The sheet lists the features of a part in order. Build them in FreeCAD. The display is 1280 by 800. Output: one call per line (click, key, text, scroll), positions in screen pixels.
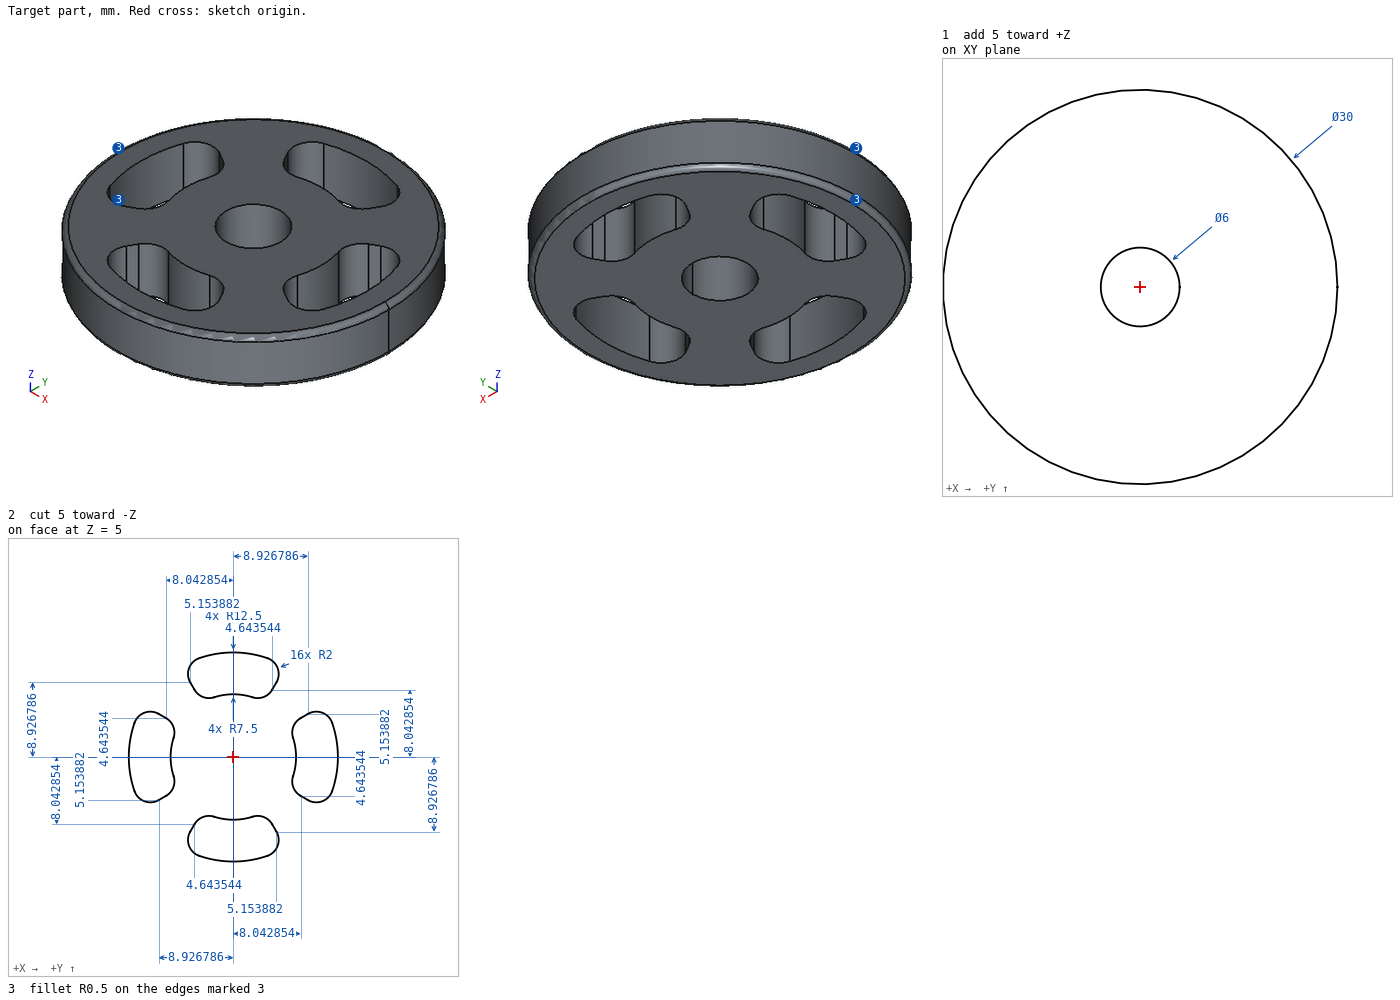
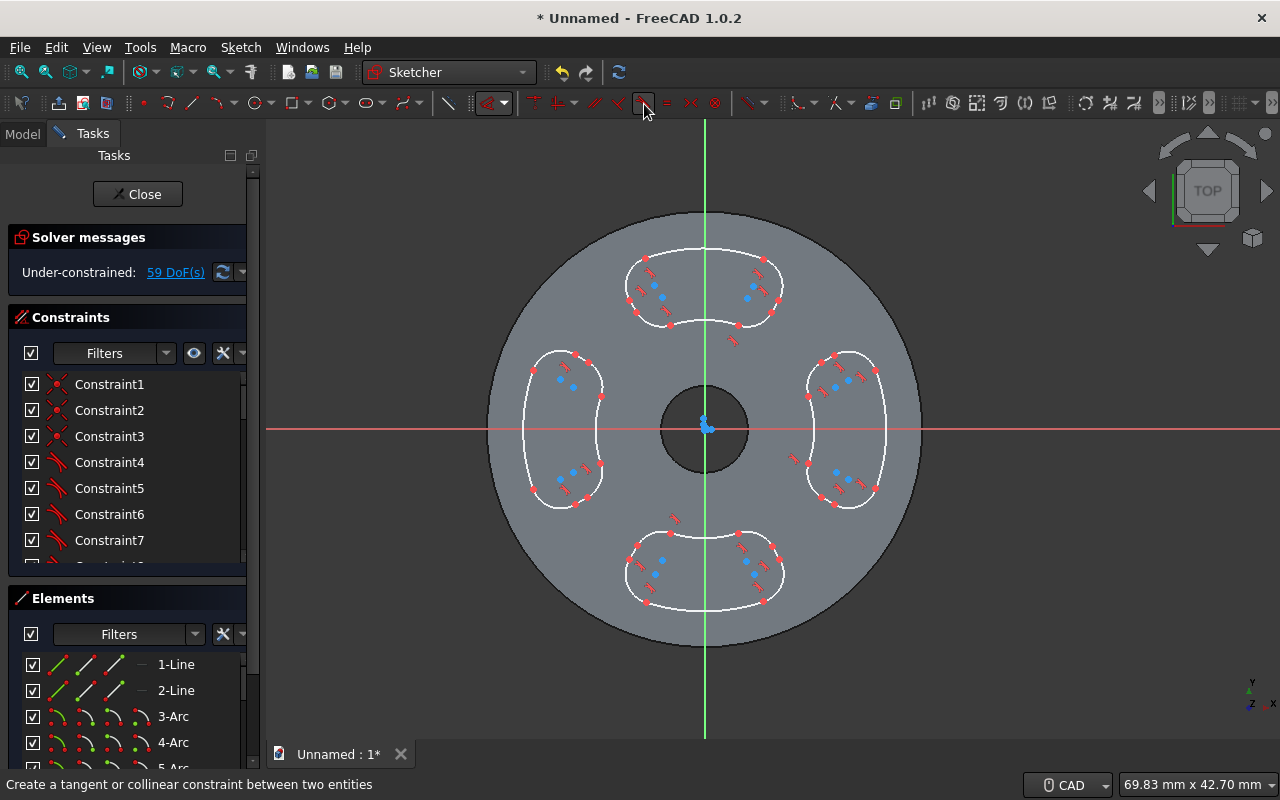
click(597, 416)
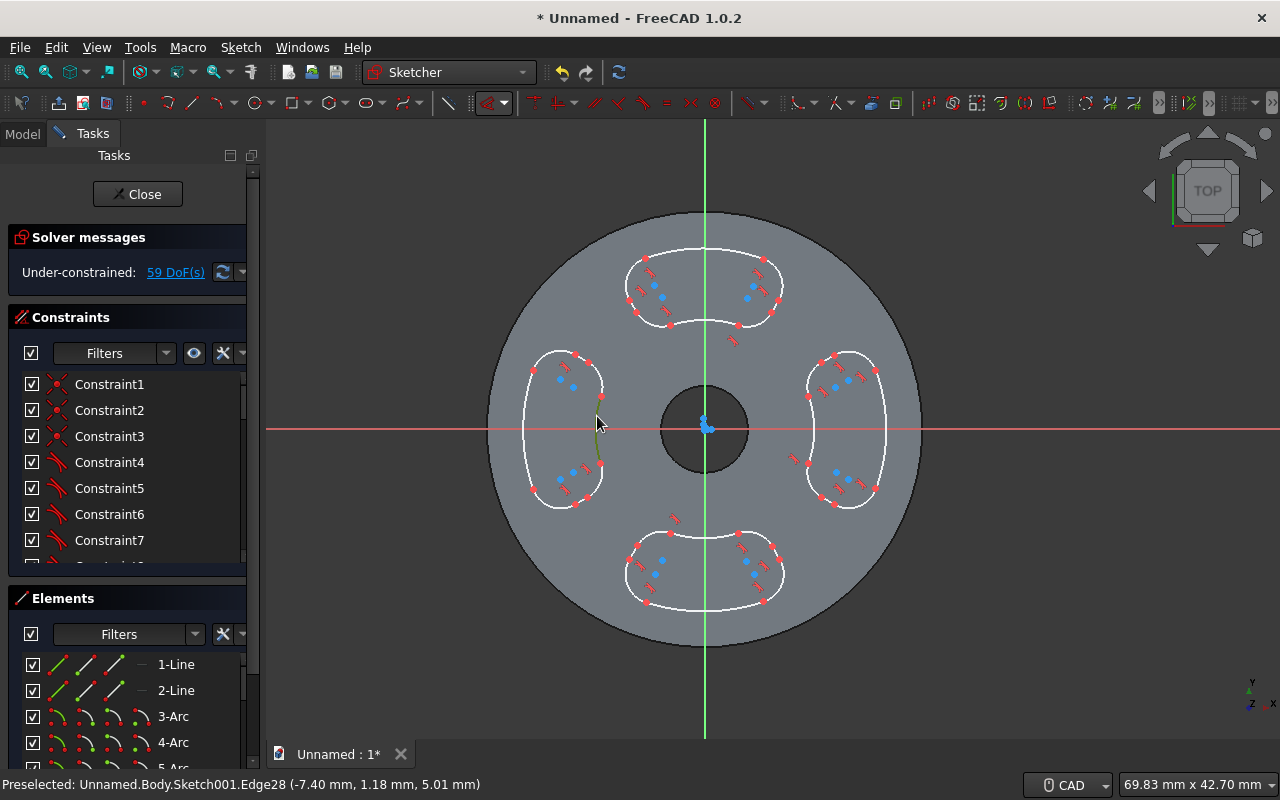
click(602, 385)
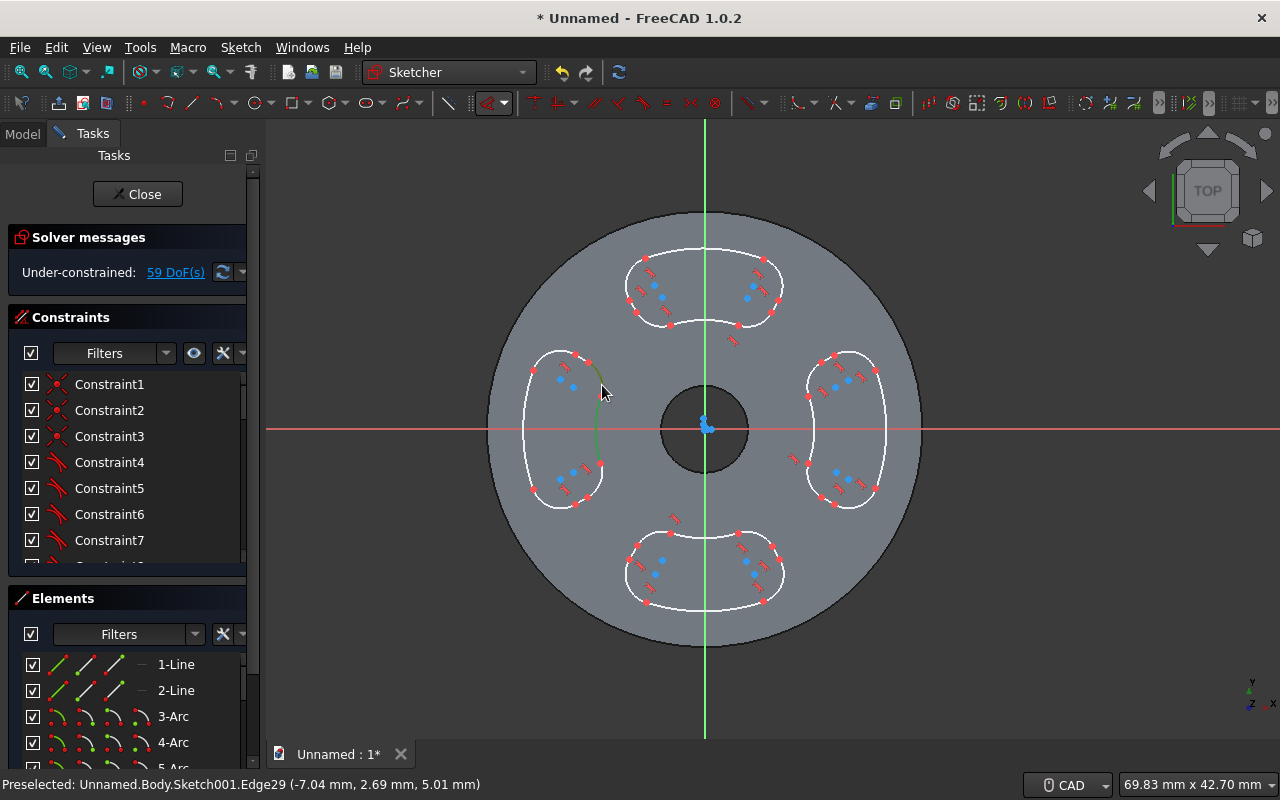
click(644, 104)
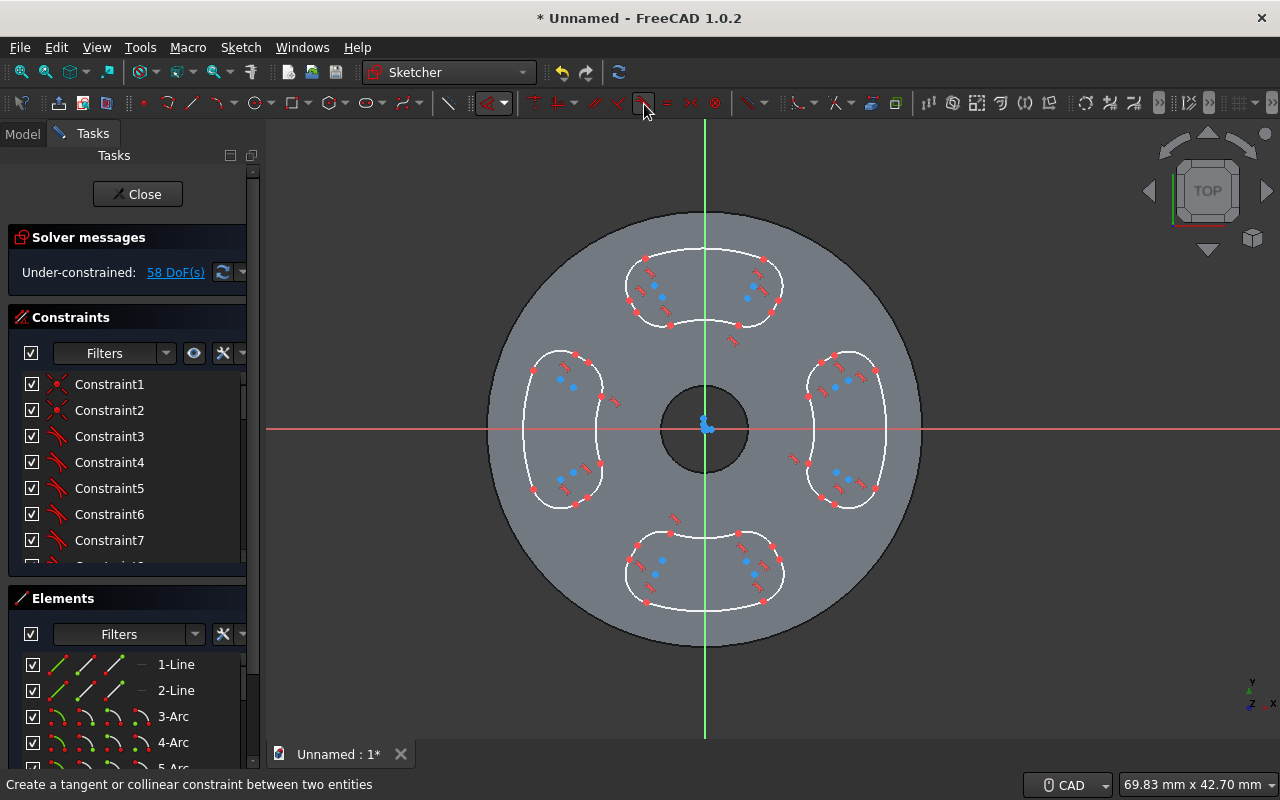
click(560, 351)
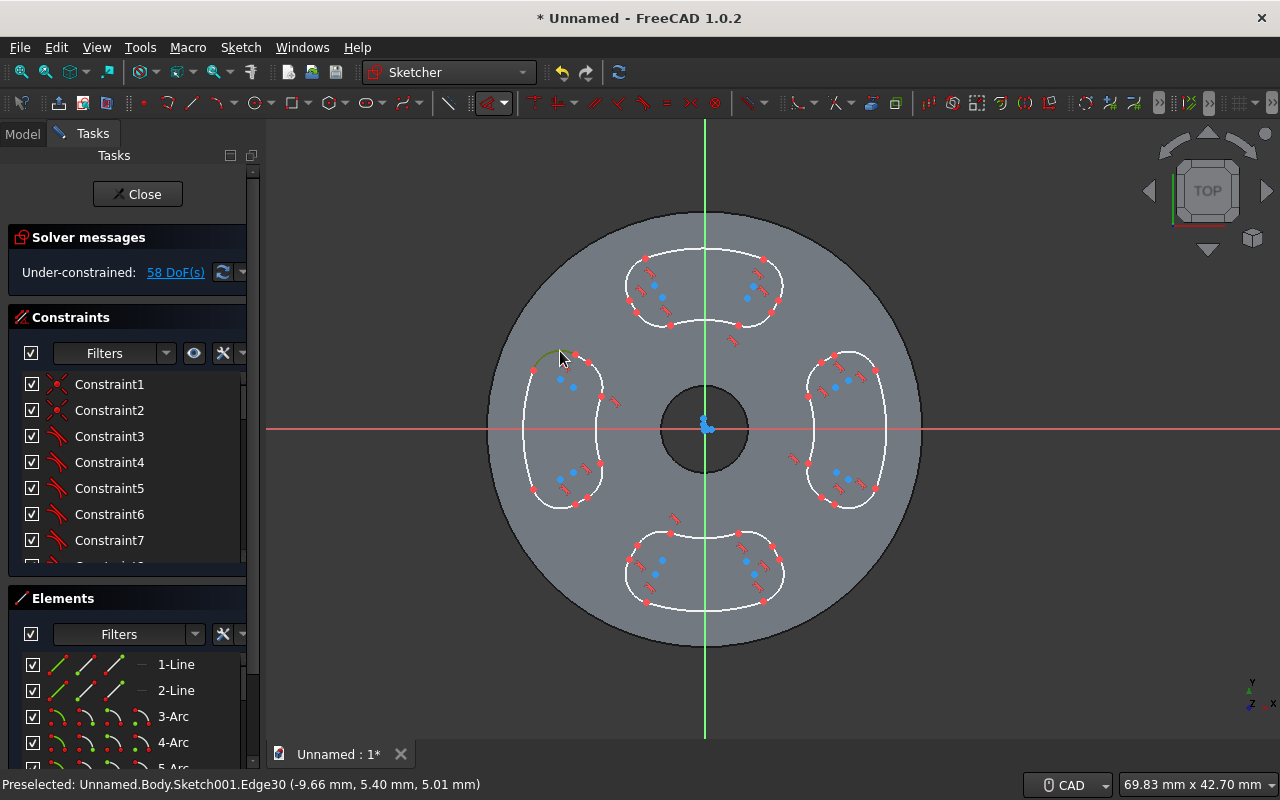
click(525, 406)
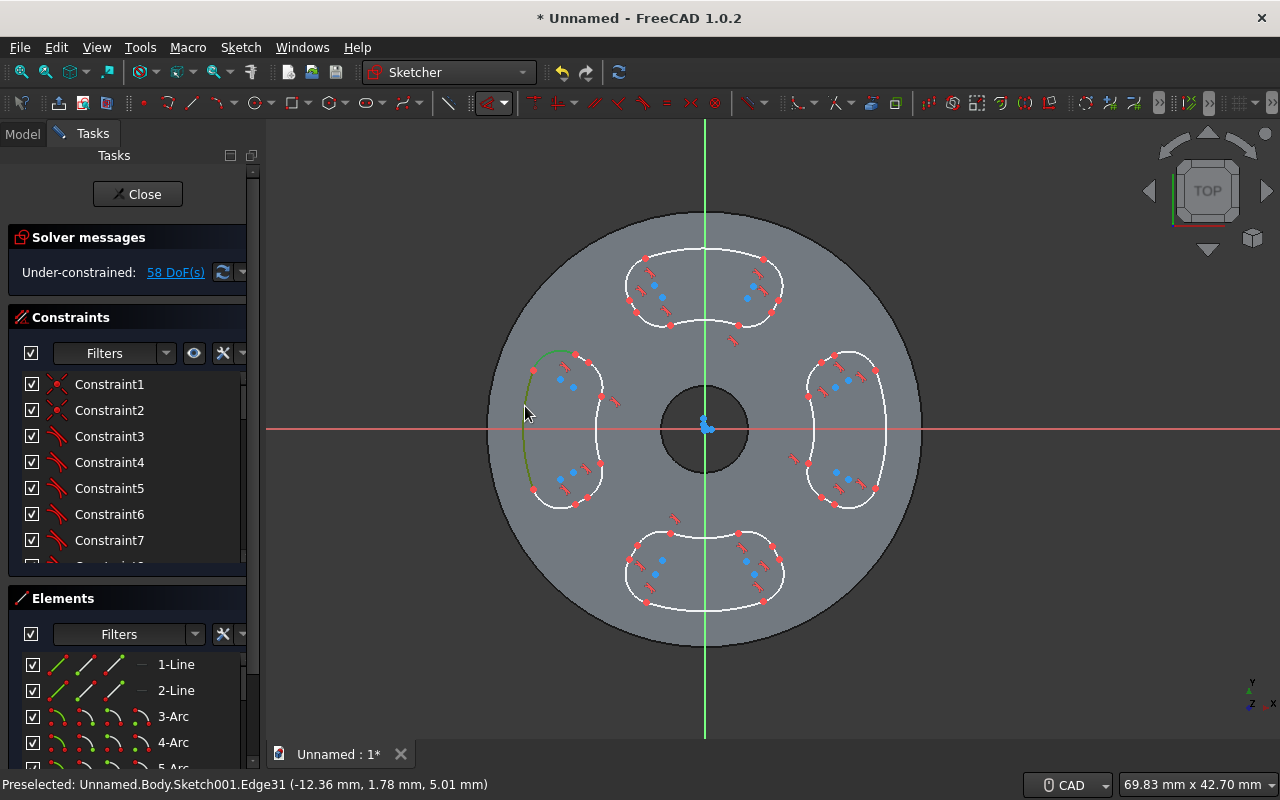
click(644, 104)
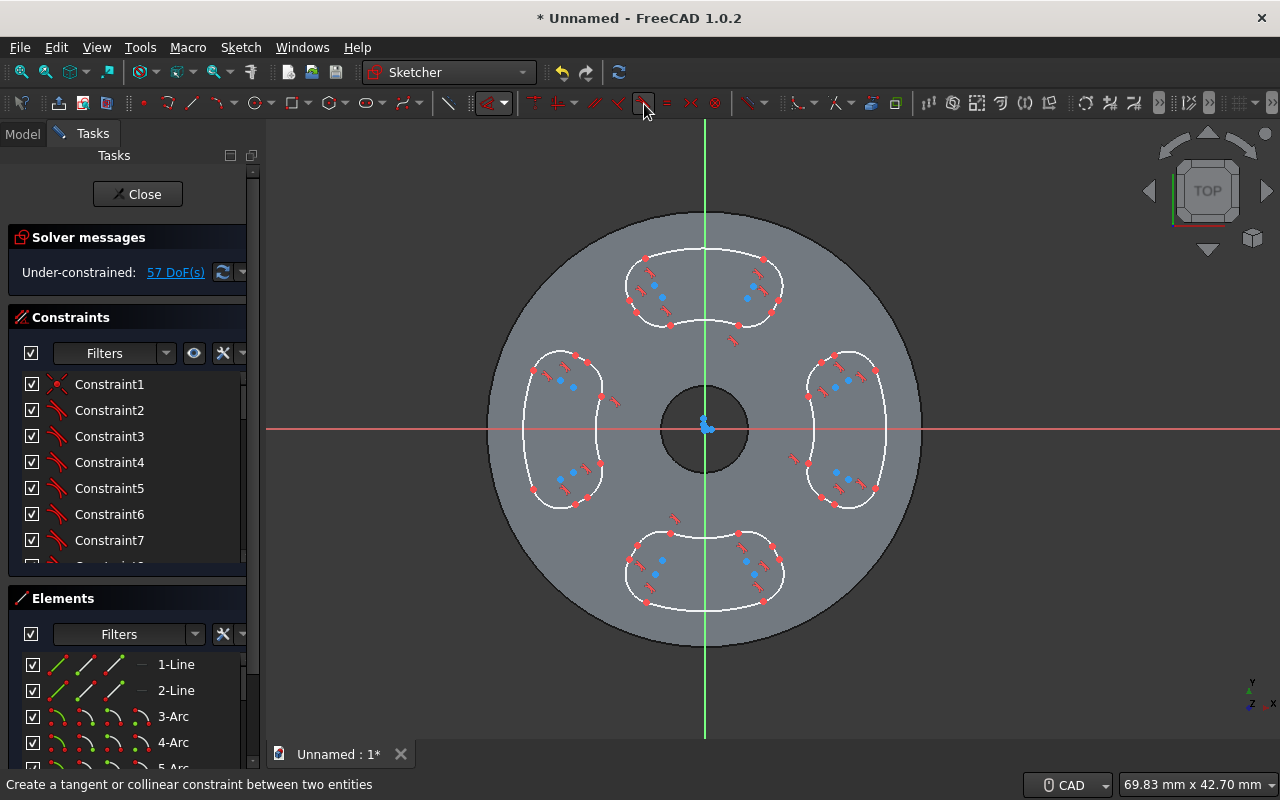
click(525, 406)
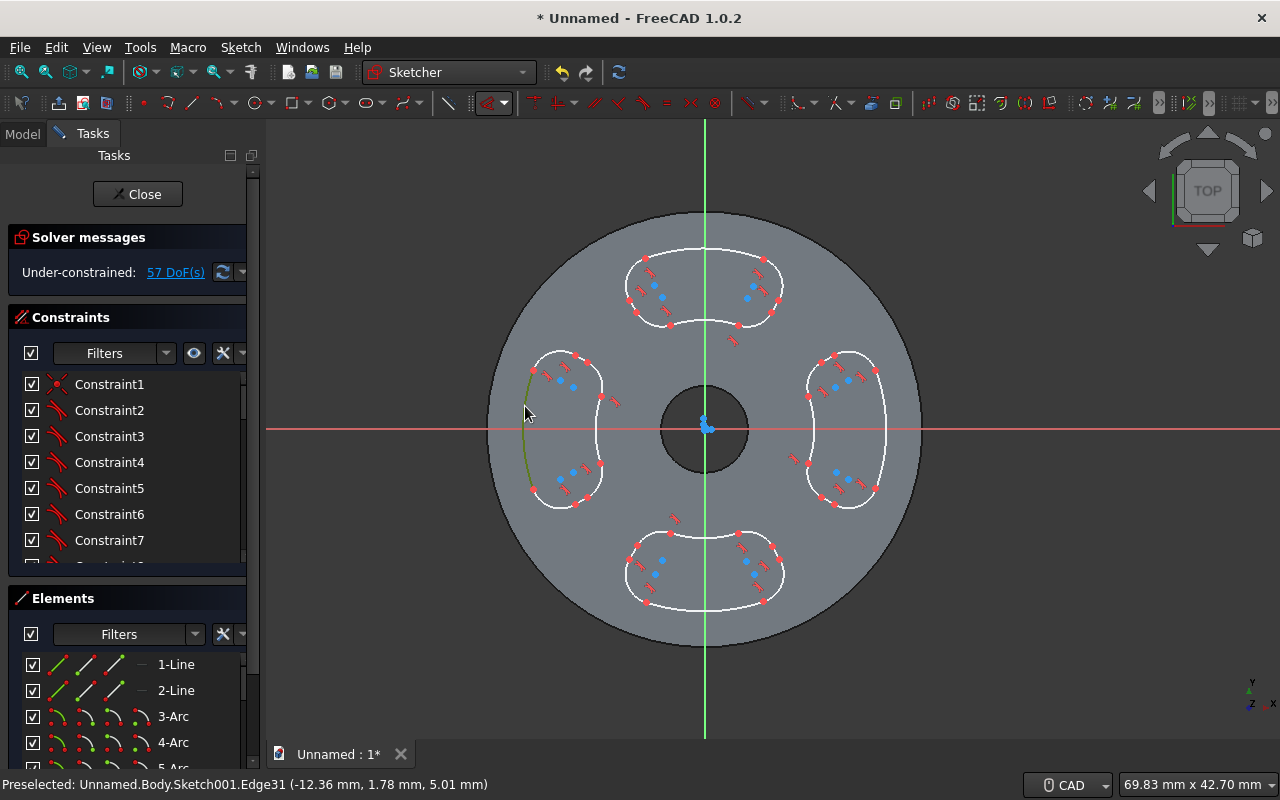
click(542, 502)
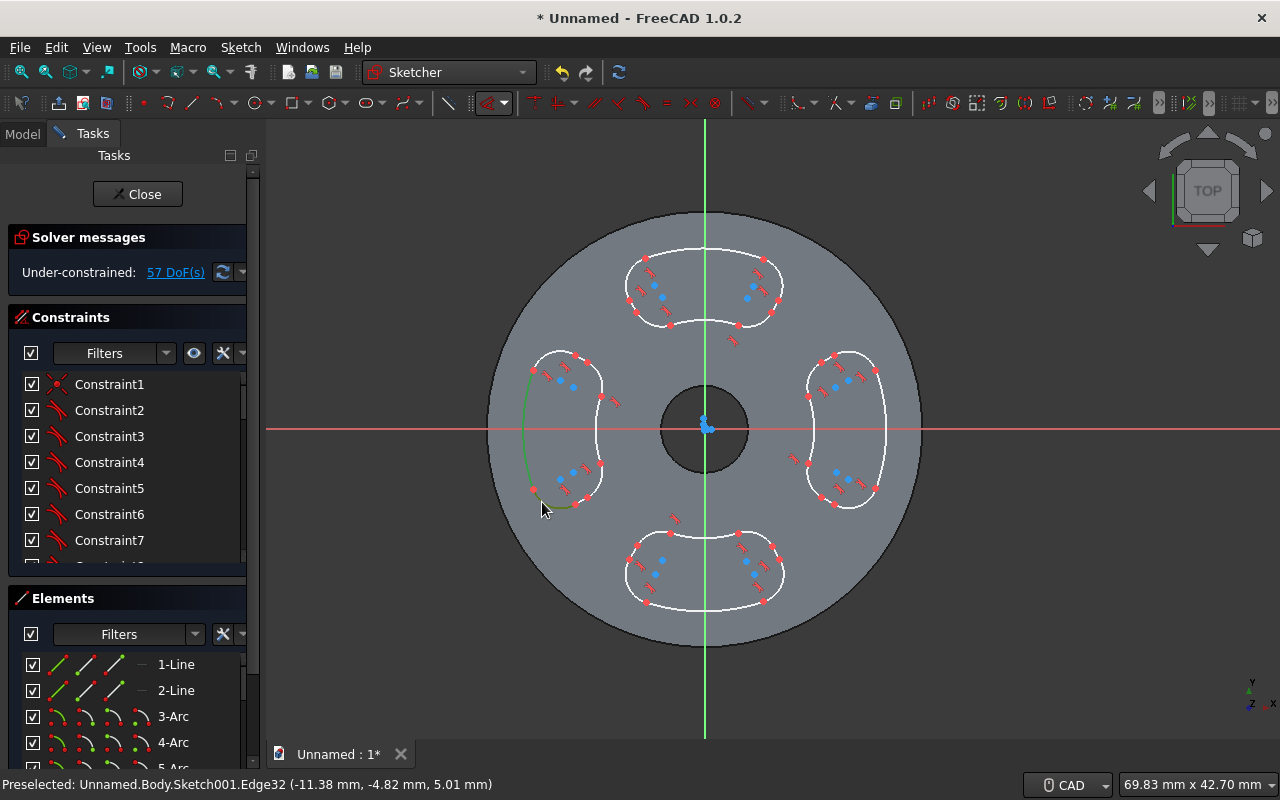
click(644, 104)